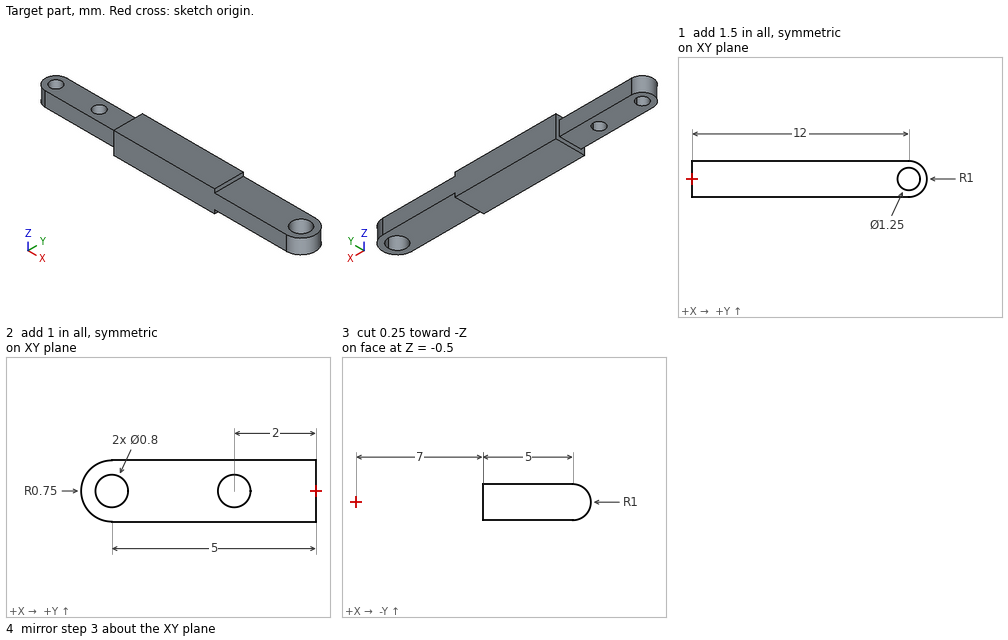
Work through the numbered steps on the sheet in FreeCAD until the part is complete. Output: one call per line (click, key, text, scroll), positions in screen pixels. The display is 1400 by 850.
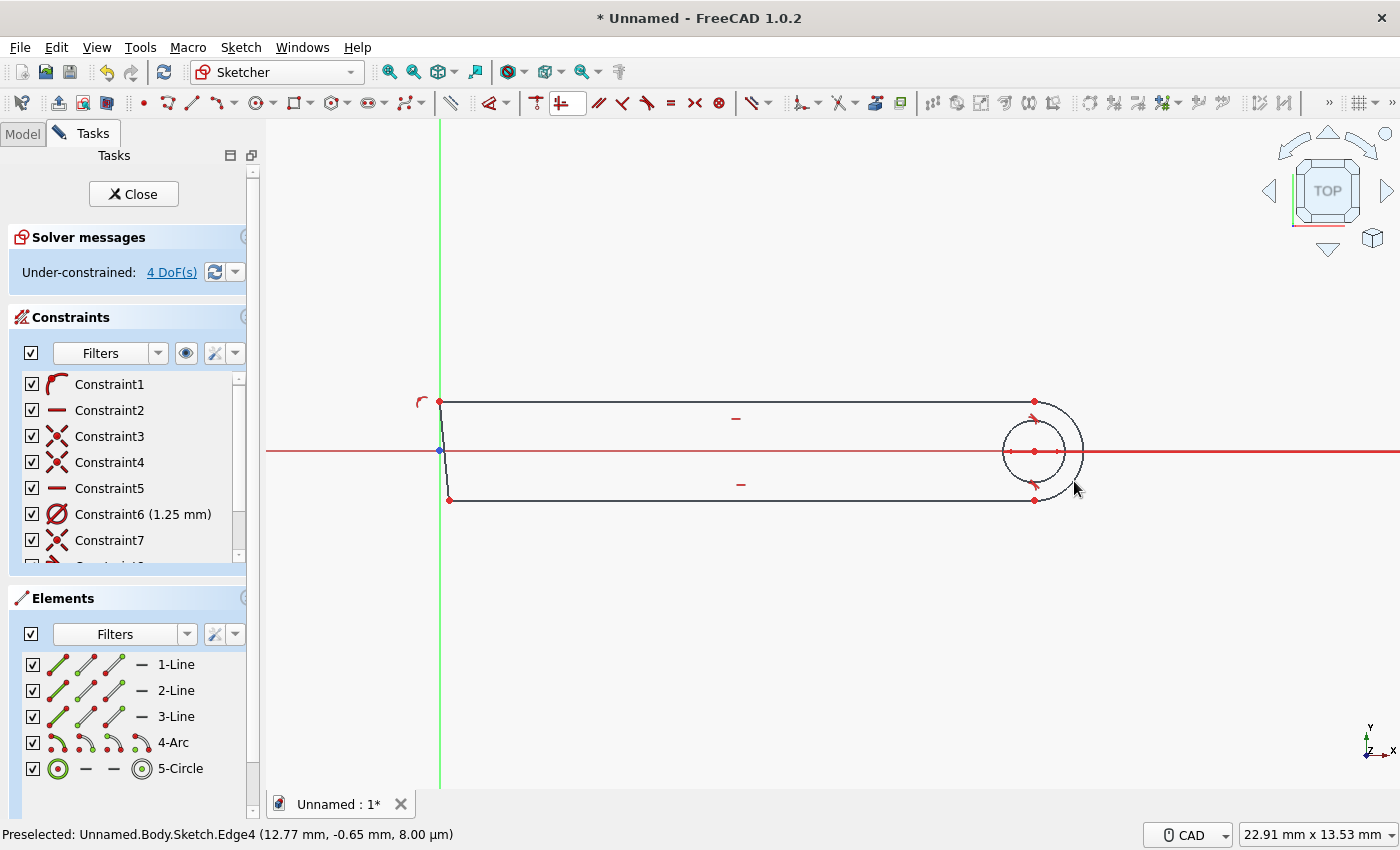
click(443, 432)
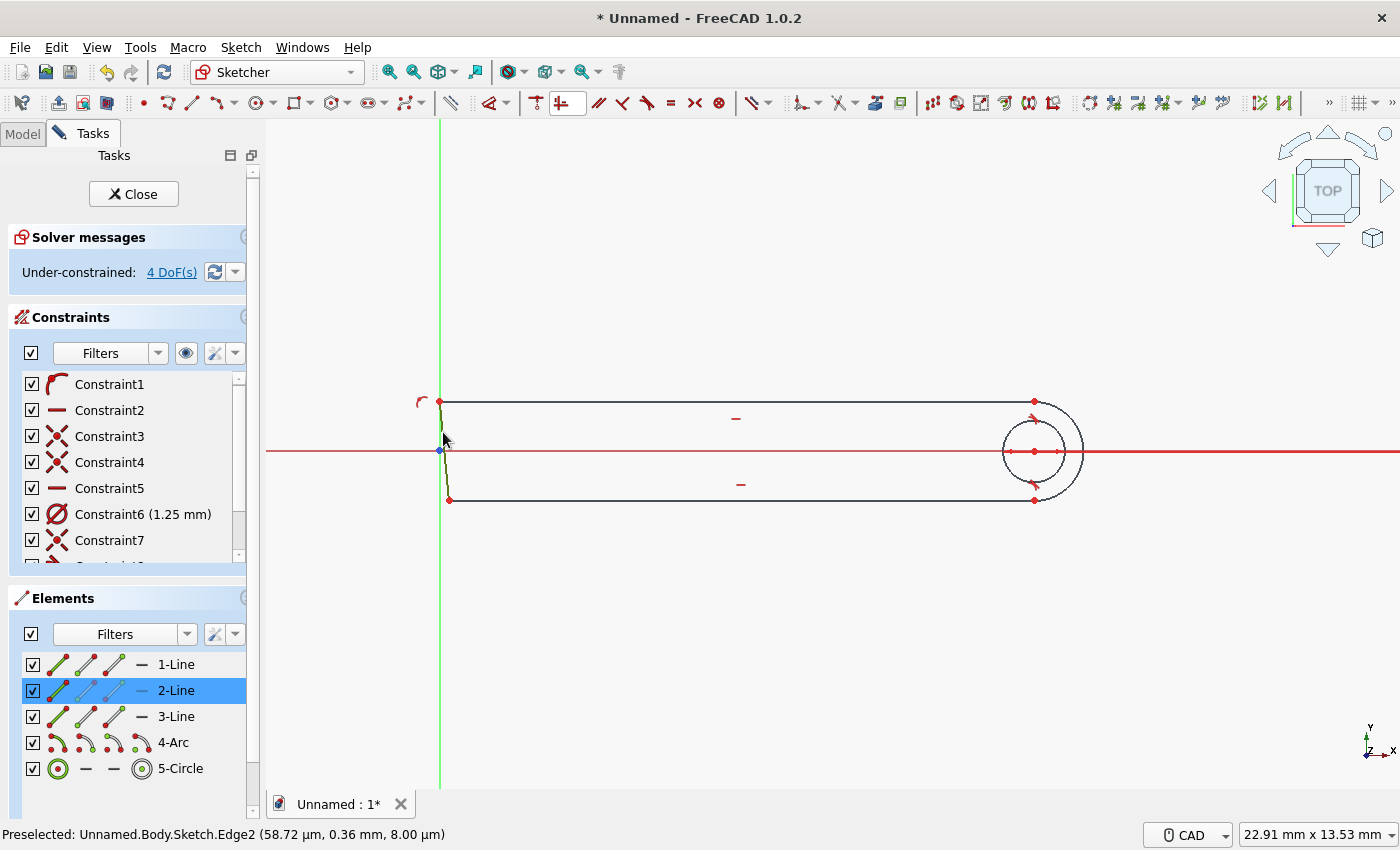
click(580, 104)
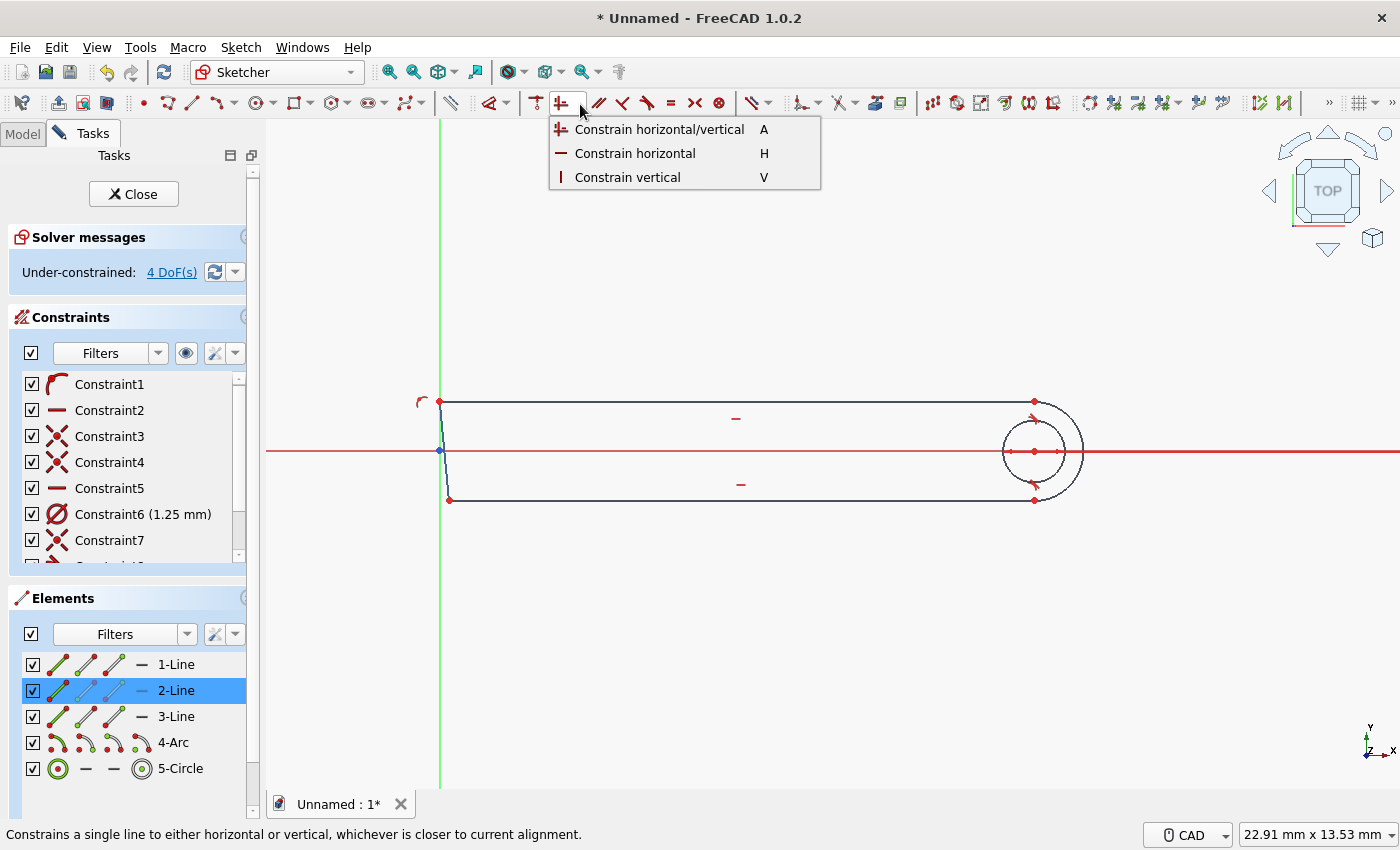
click(685, 177)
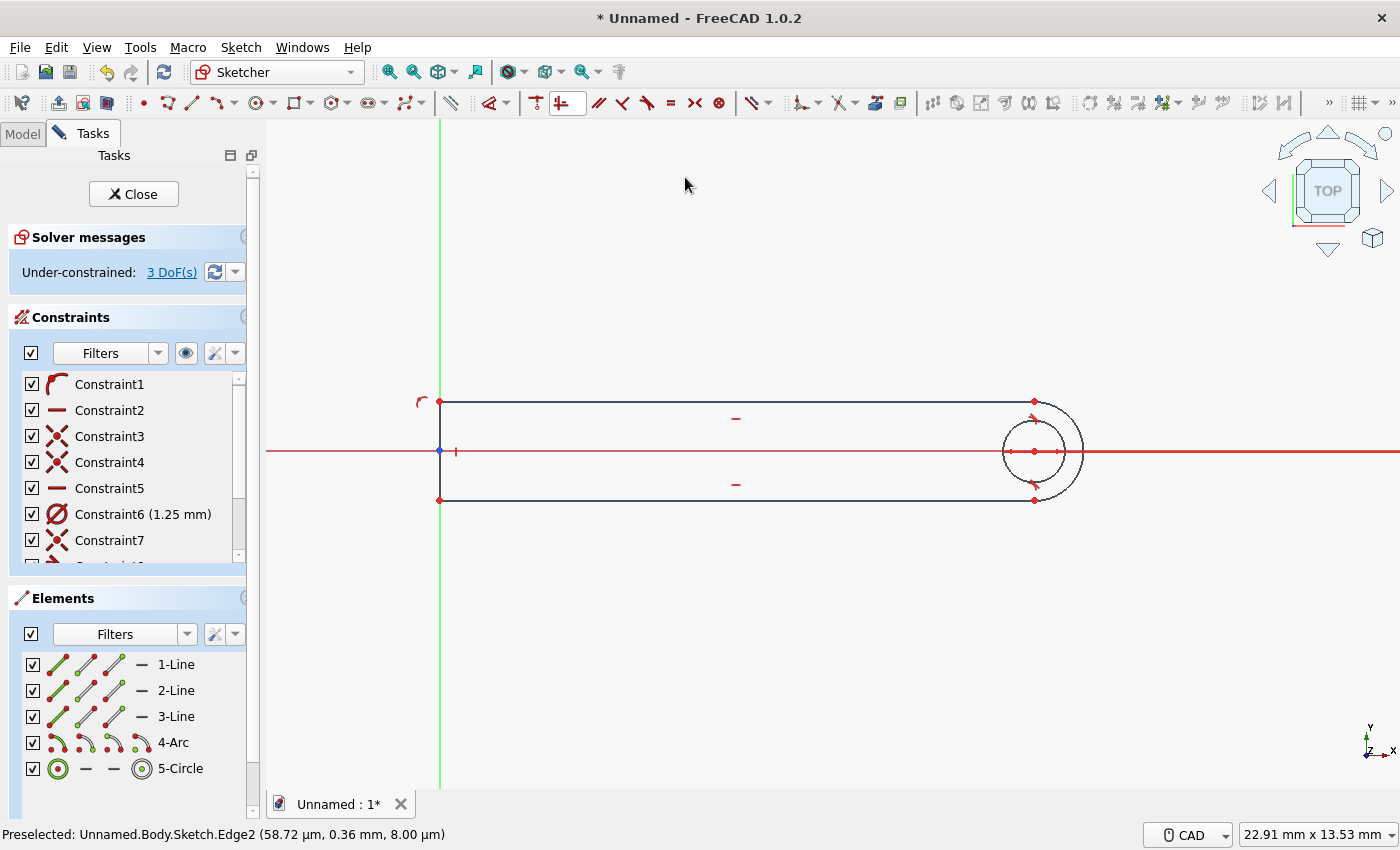
click(1034, 452)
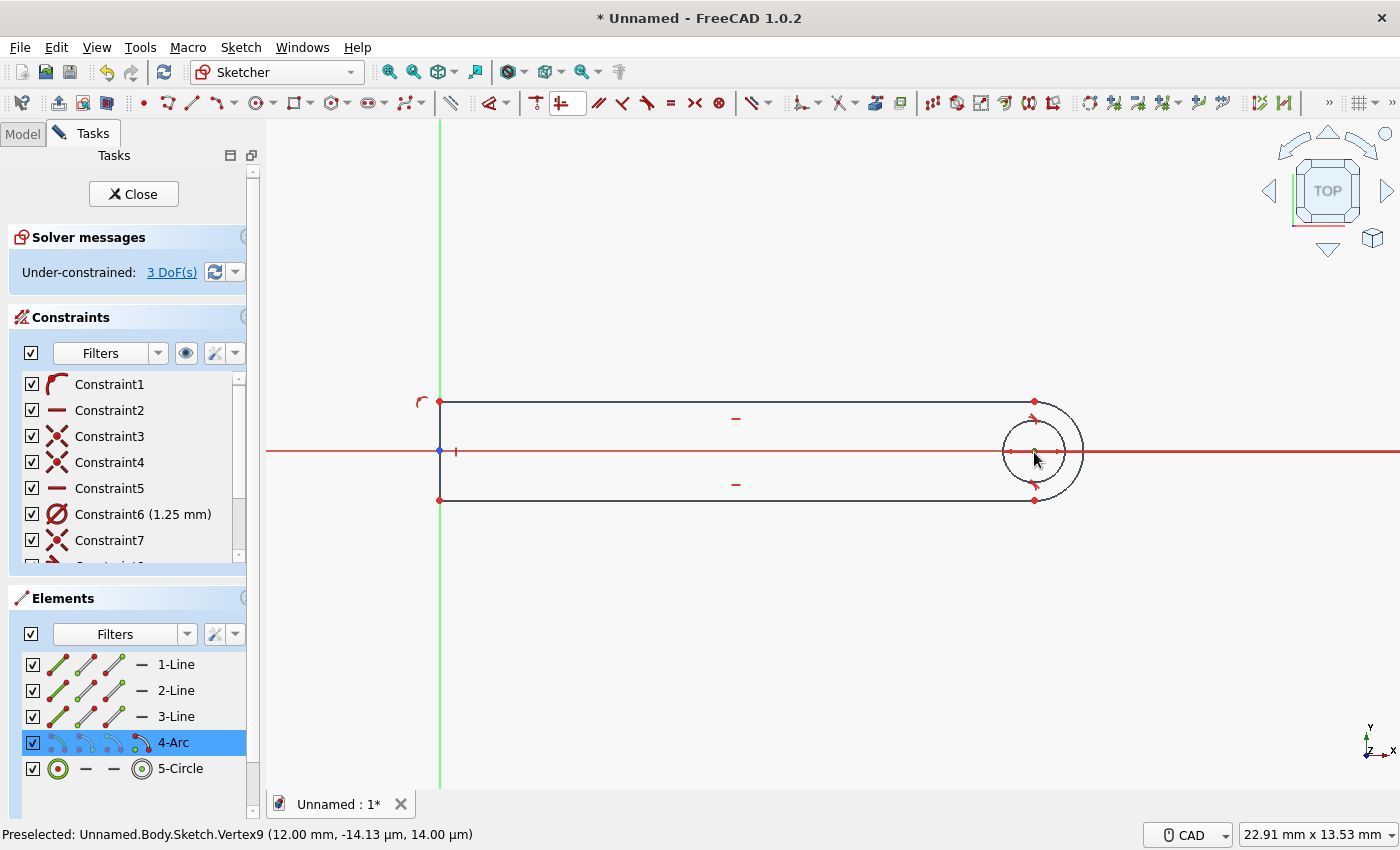
click(361, 451)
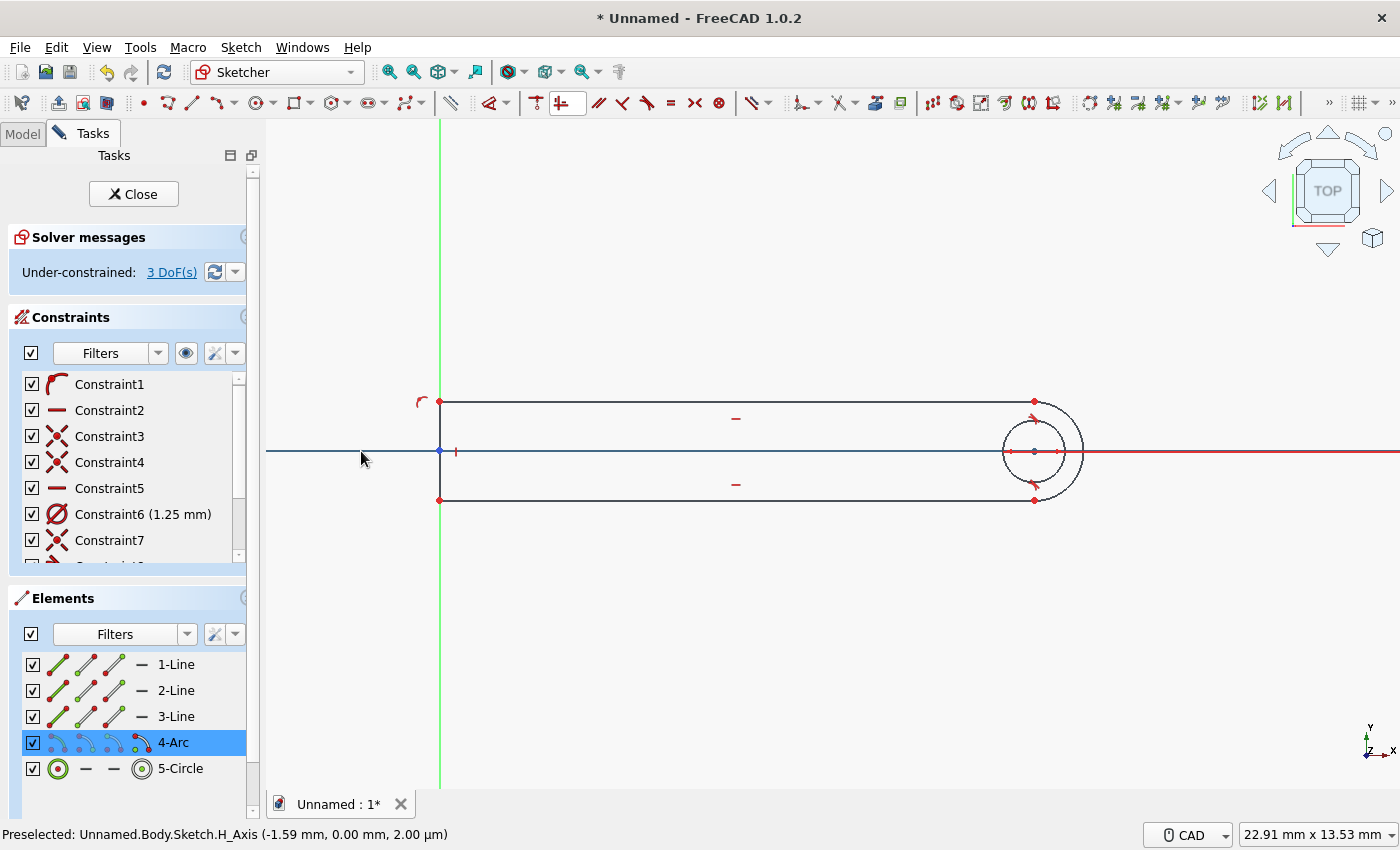
click(536, 104)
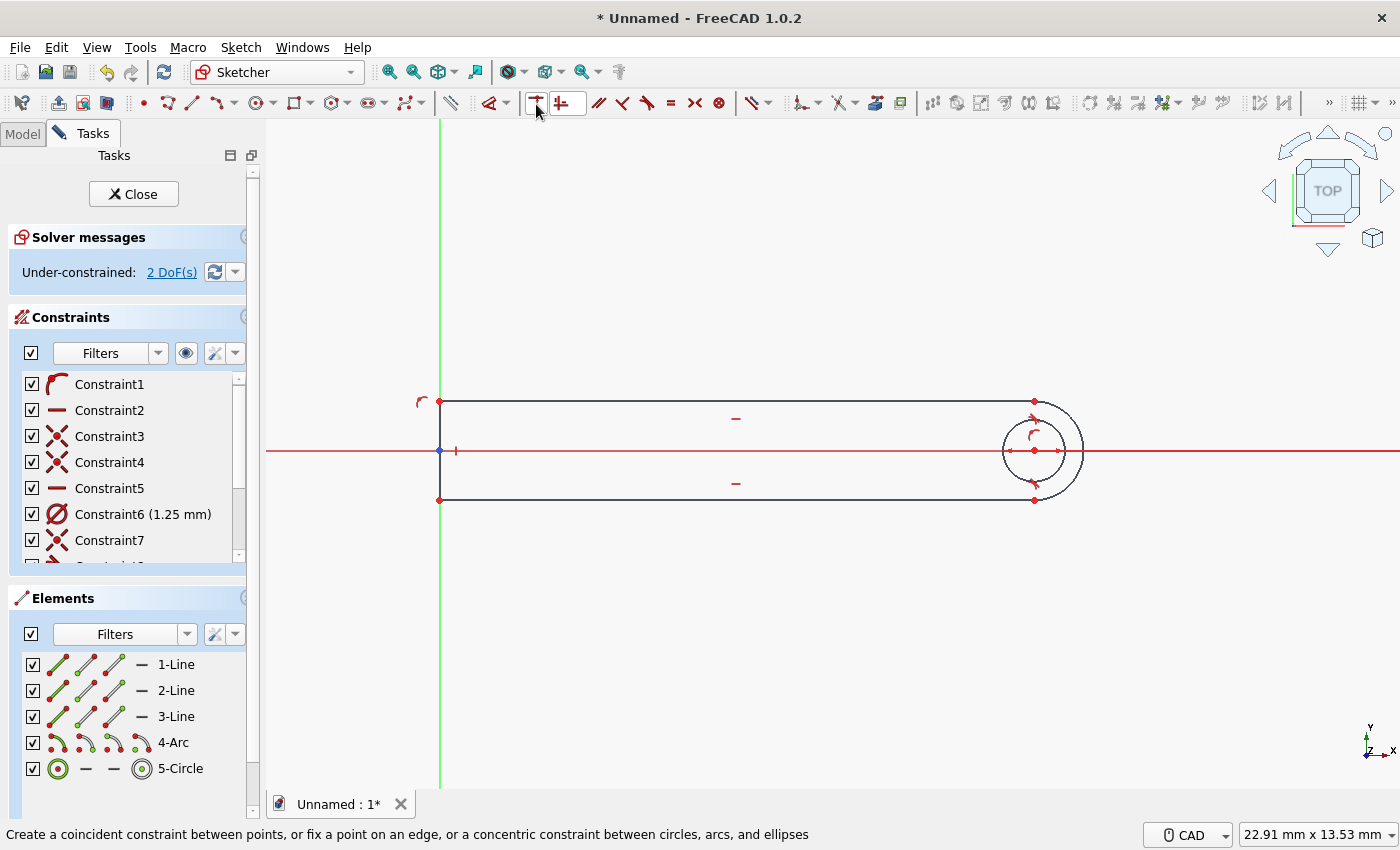
click(490, 104)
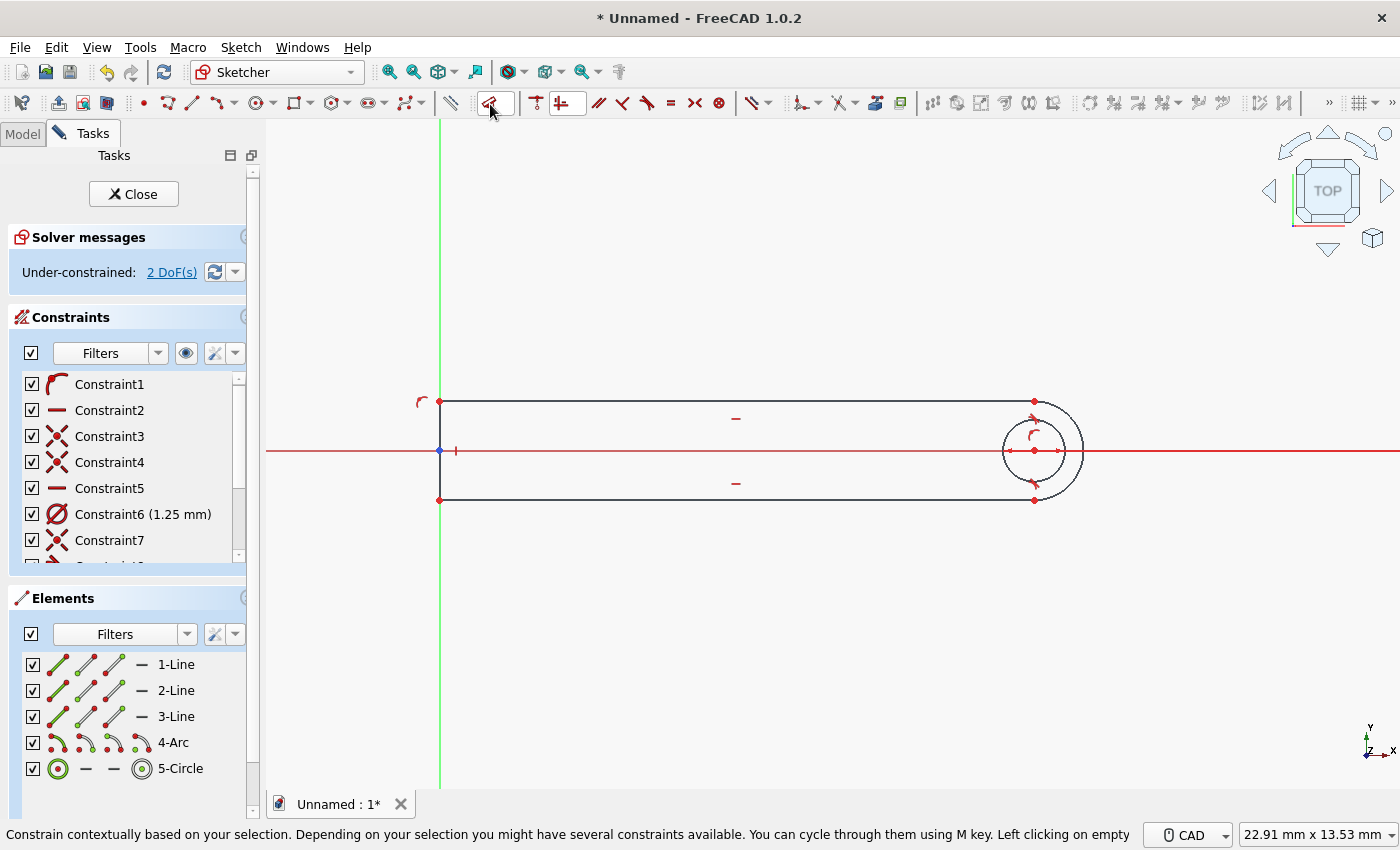
click(1074, 480)
click(1100, 499)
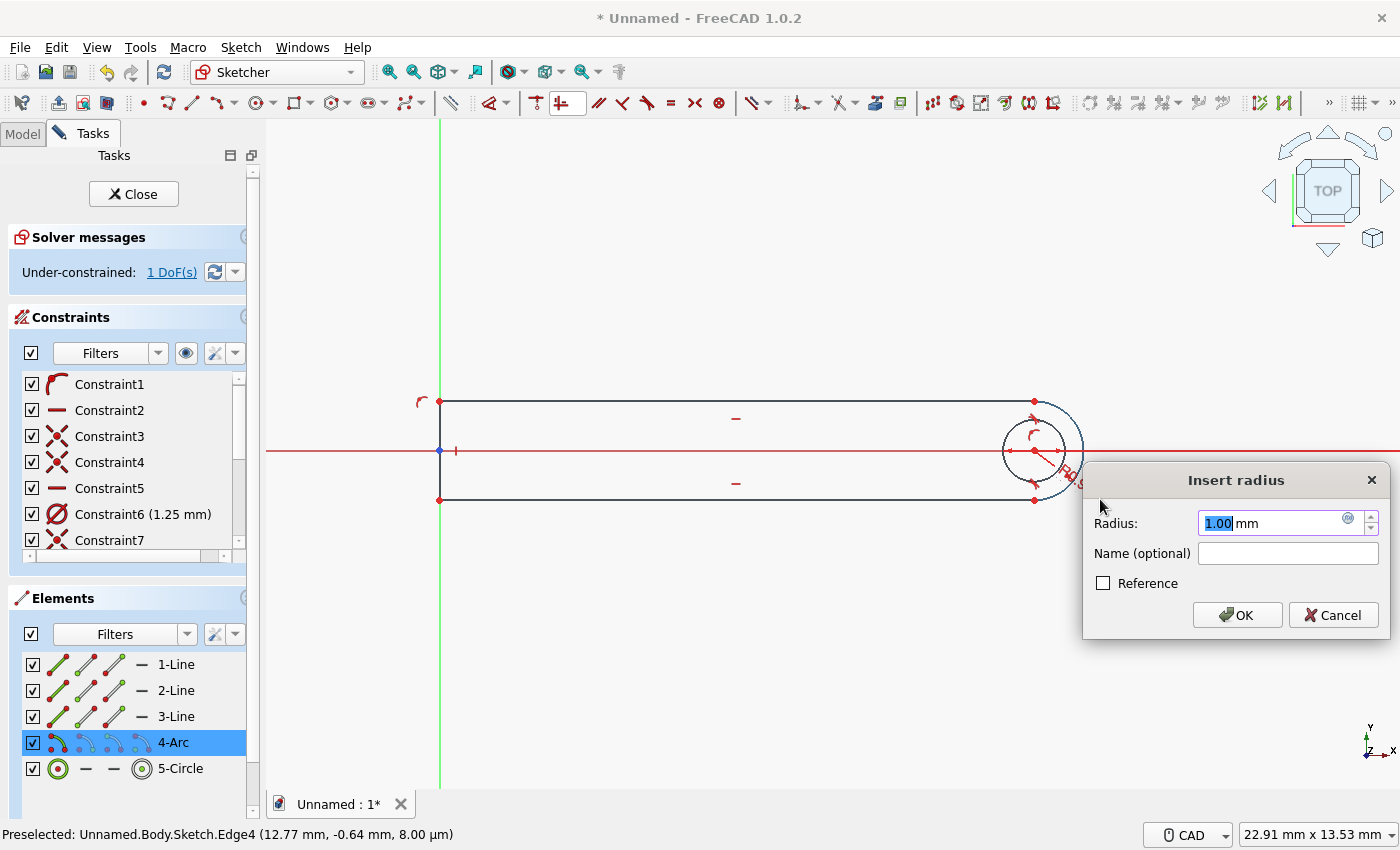
text(1)
key(Return)